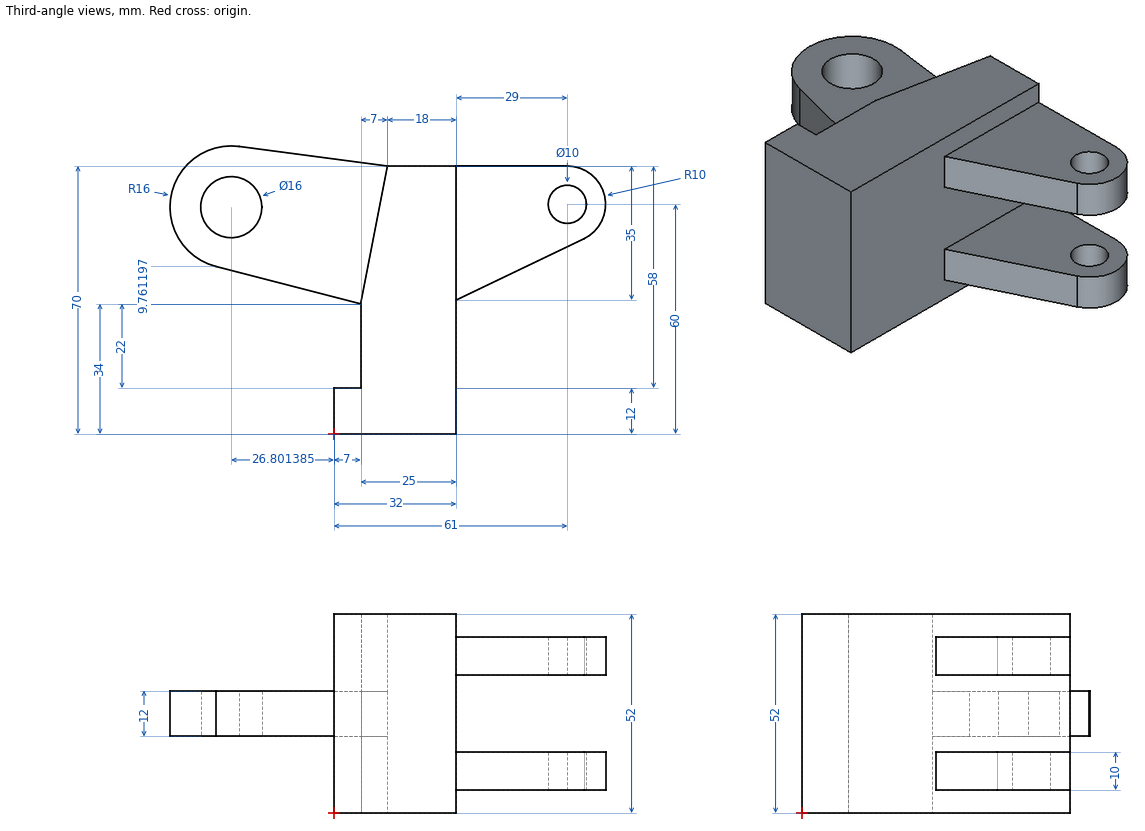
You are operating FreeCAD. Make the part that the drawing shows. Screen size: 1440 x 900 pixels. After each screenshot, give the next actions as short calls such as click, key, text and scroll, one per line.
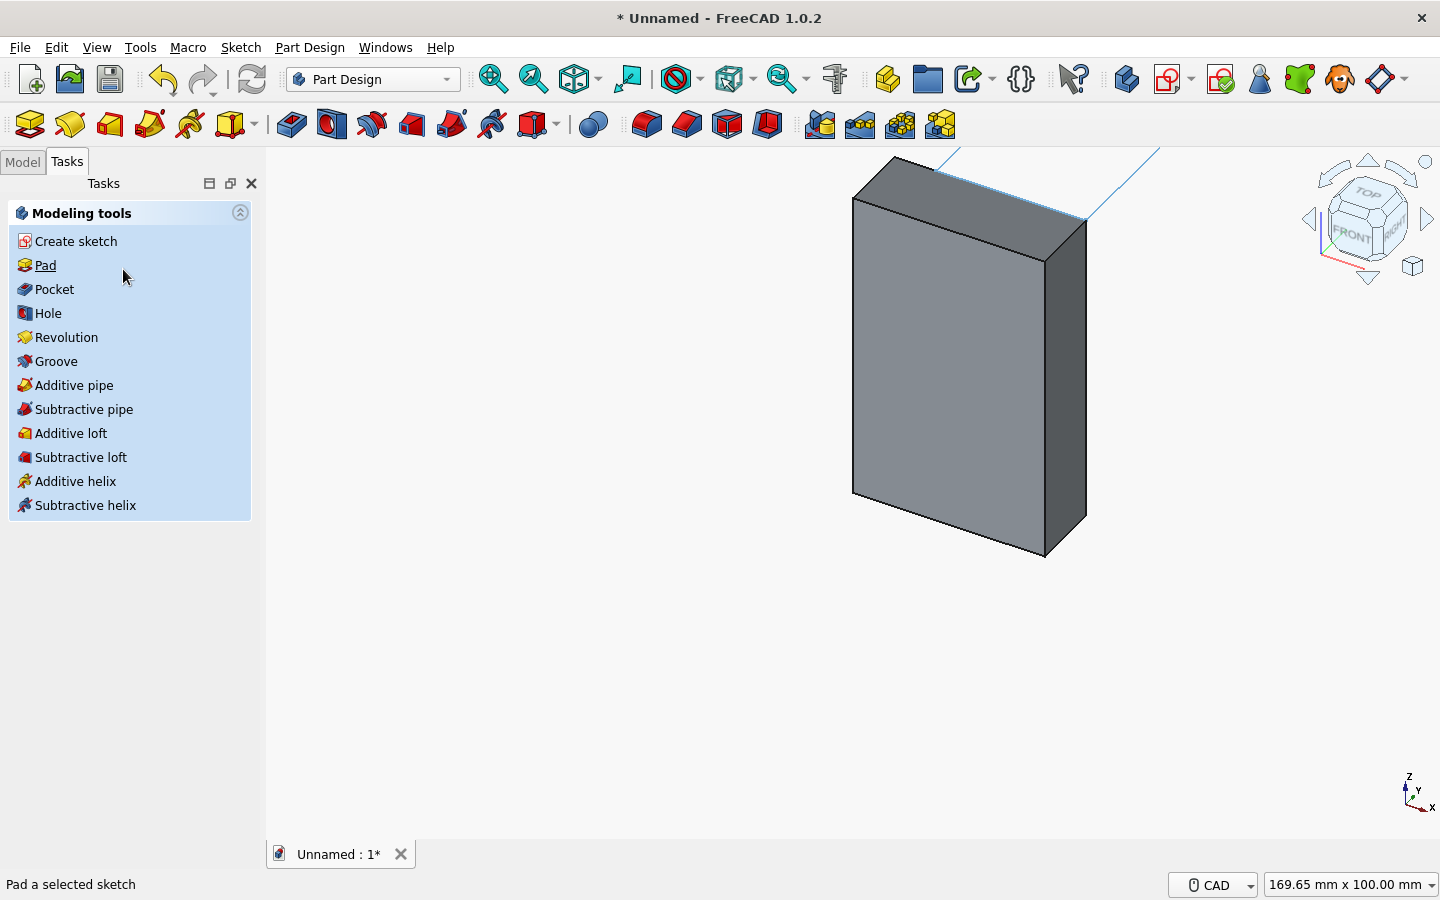
click(30, 124)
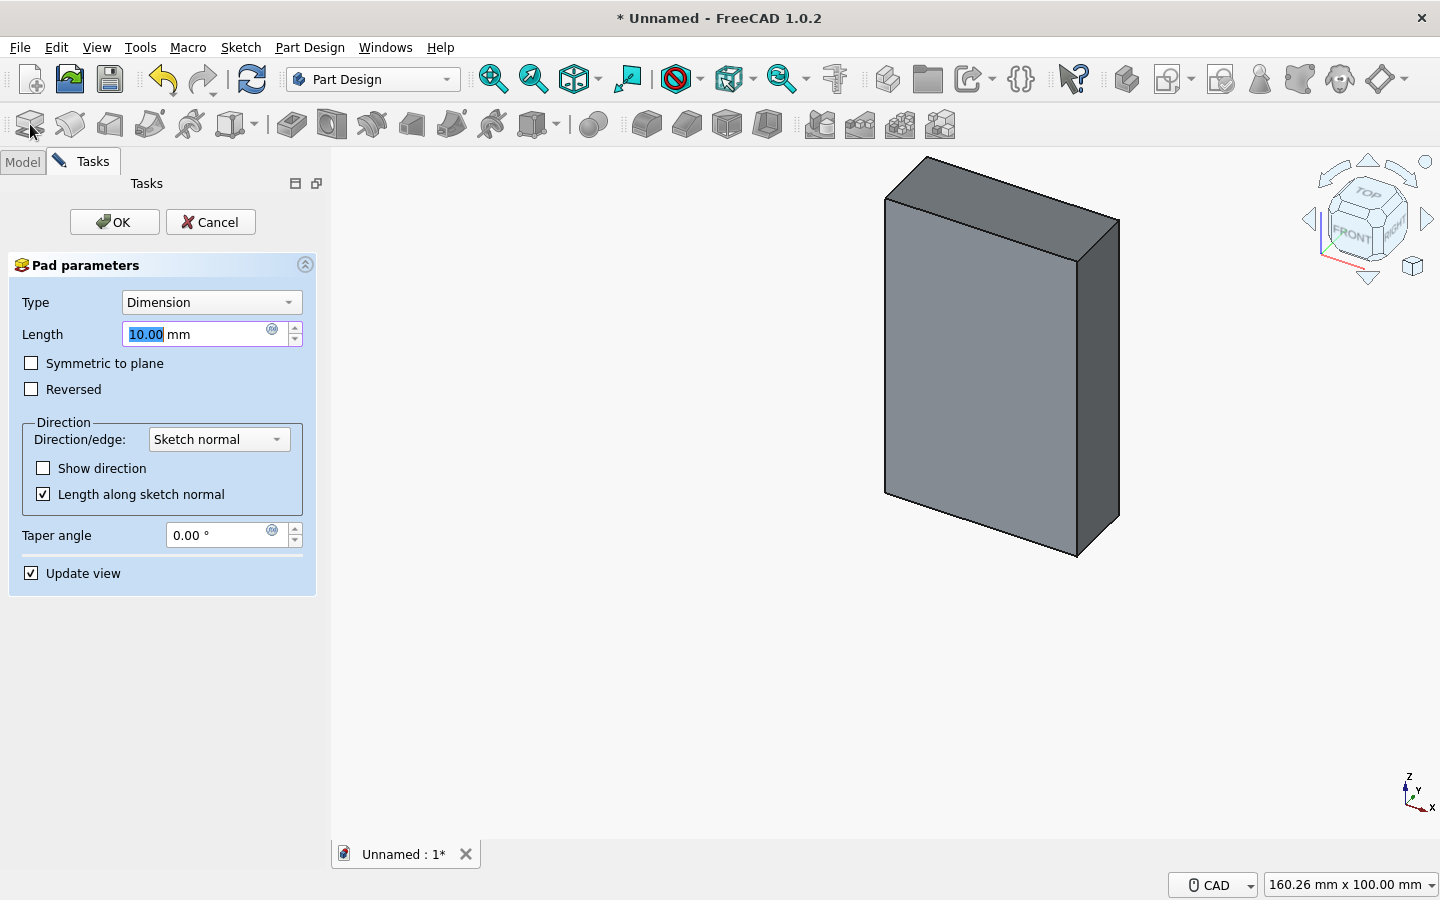
text(52)
key(Tab)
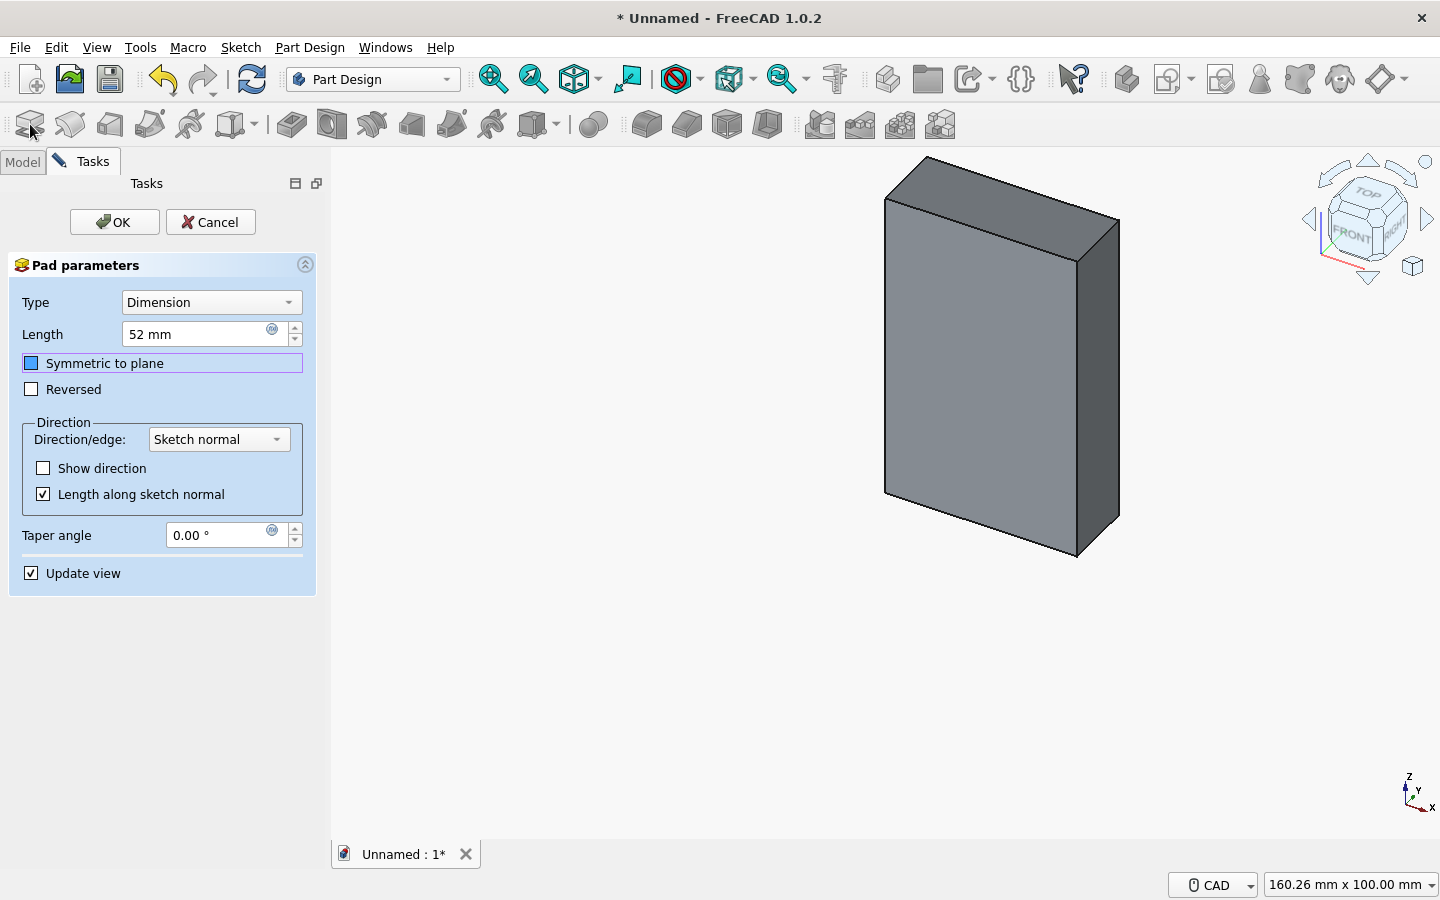
click(30, 389)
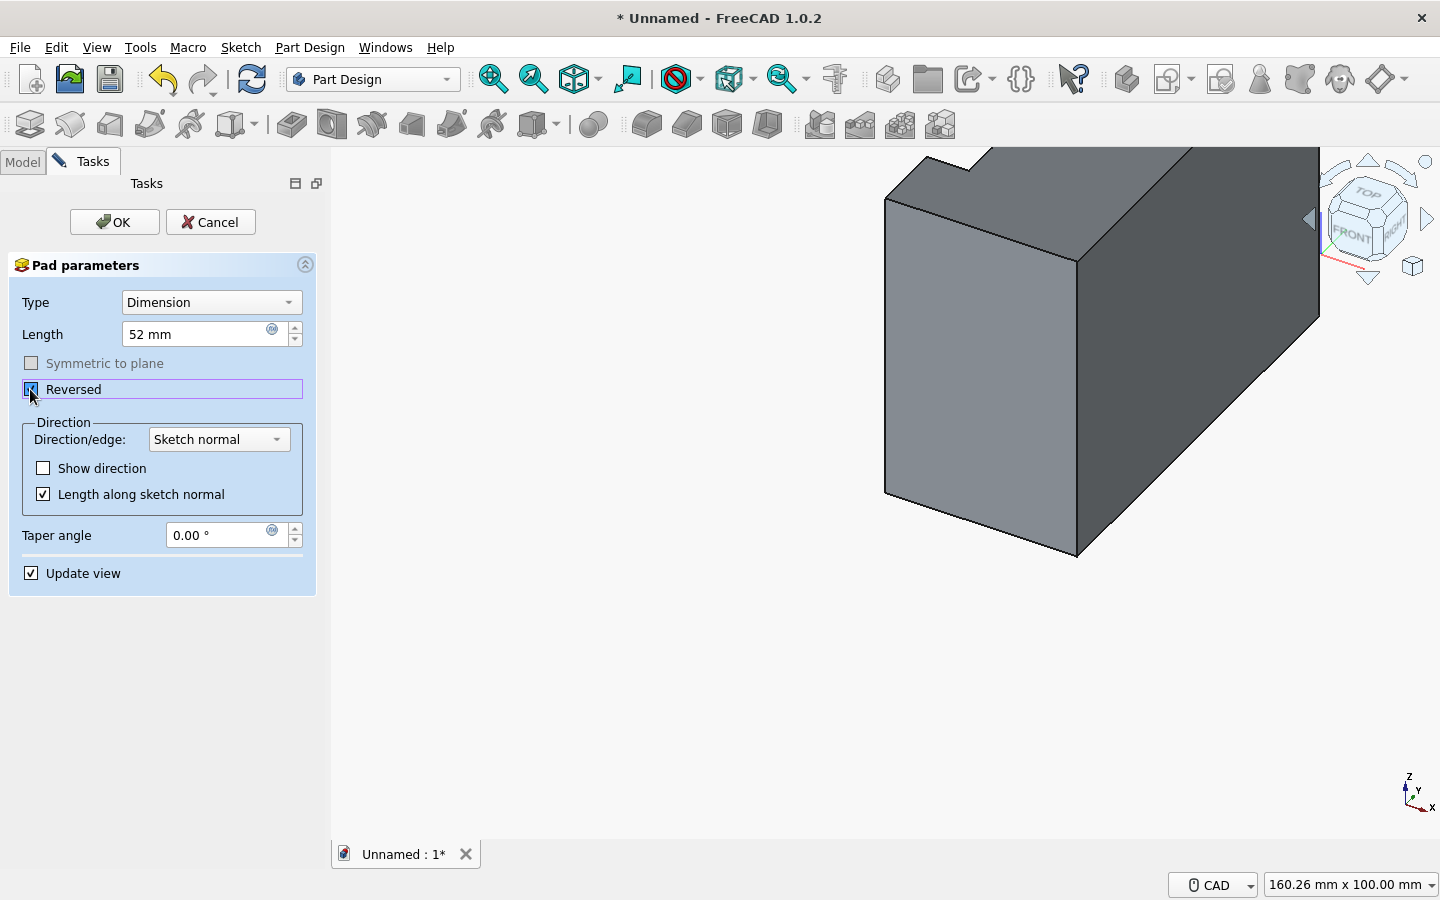
click(115, 222)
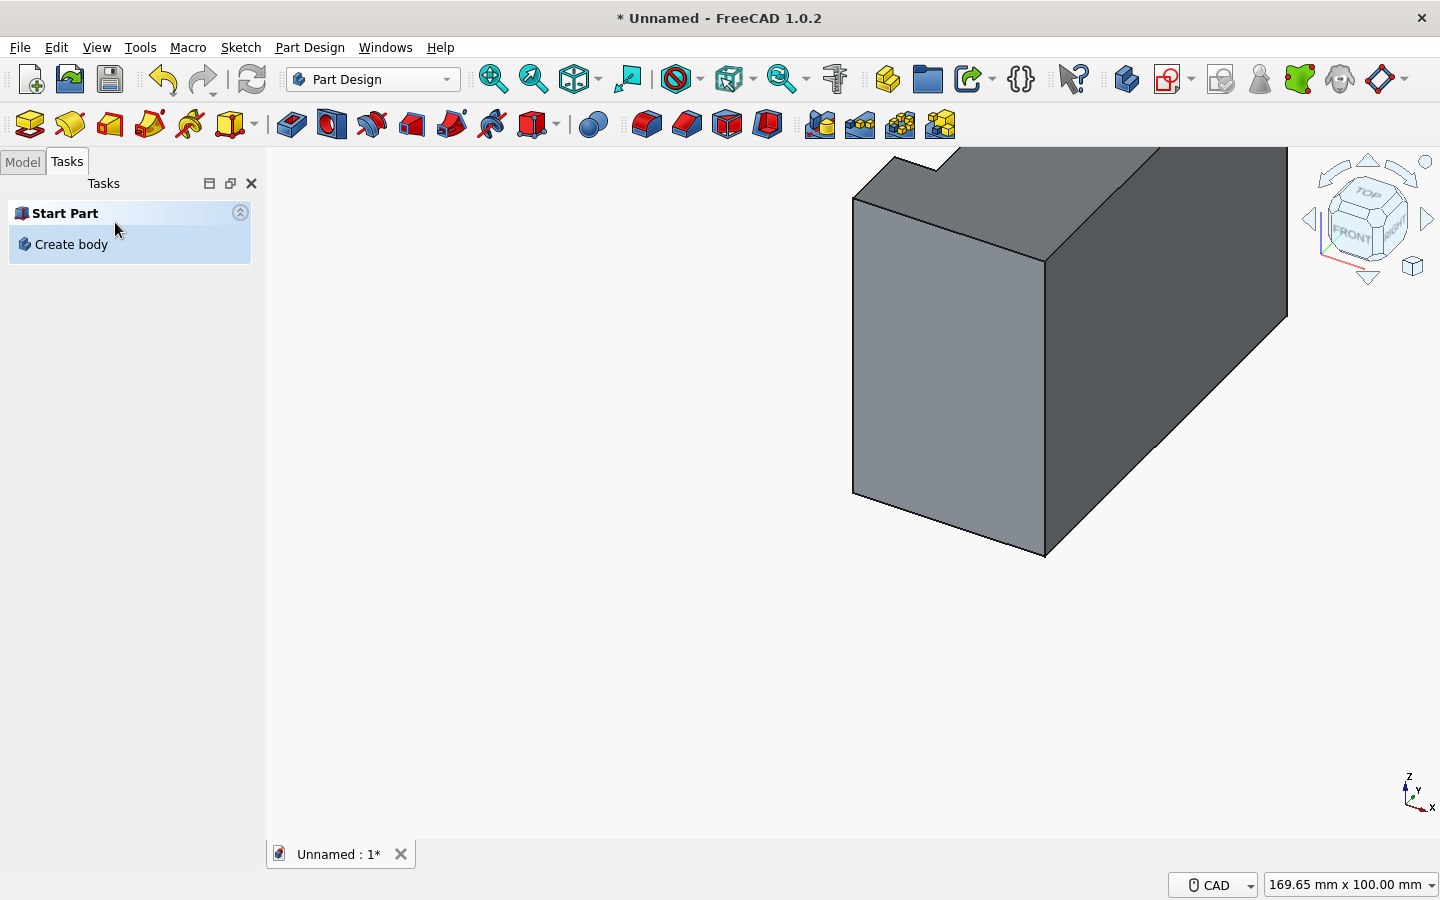
key(v)
key(f)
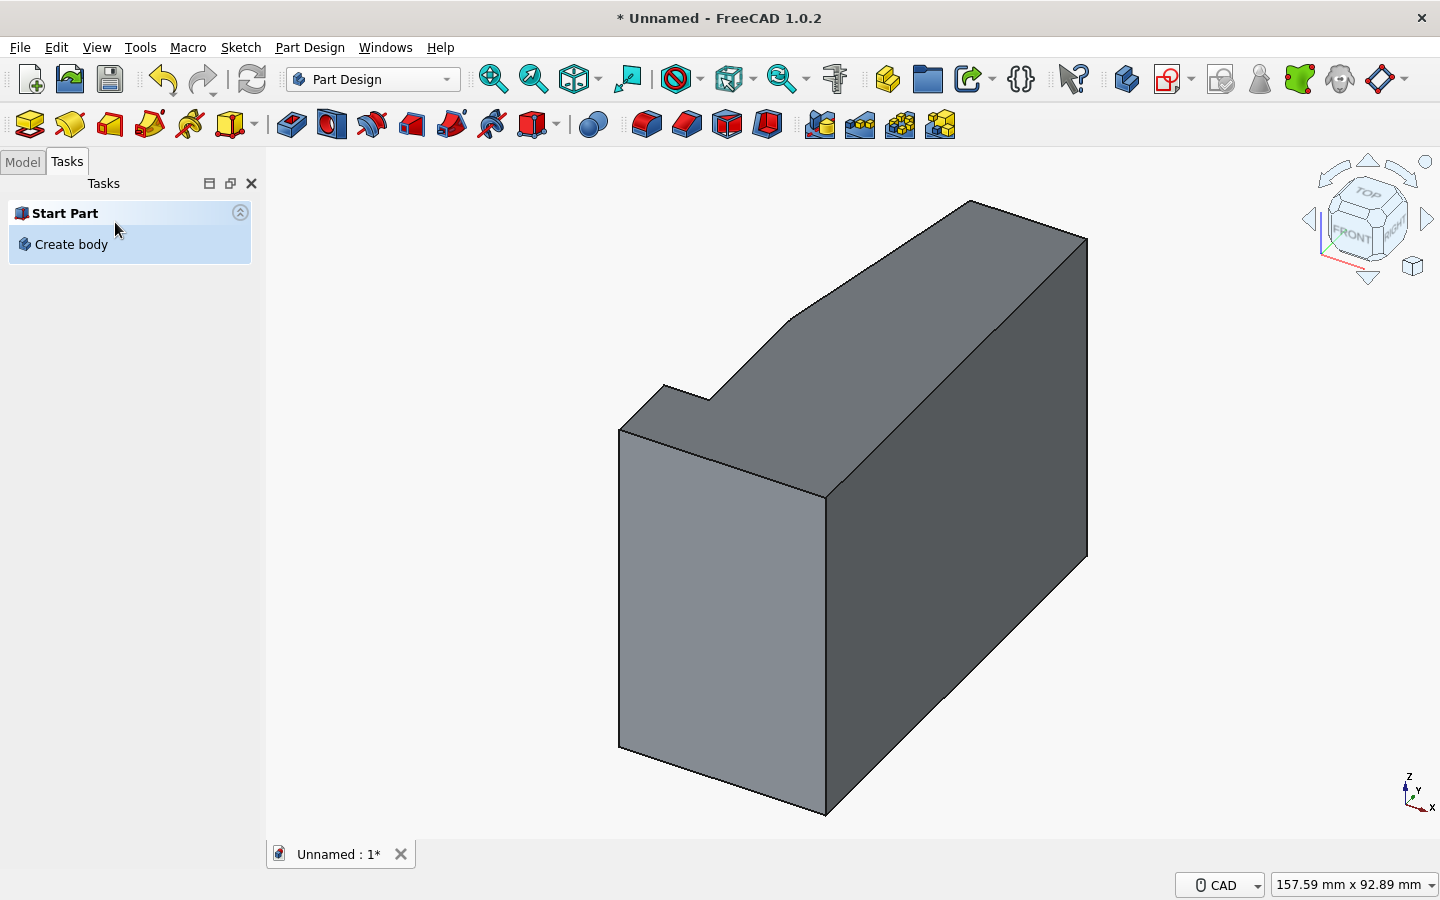
click(23, 161)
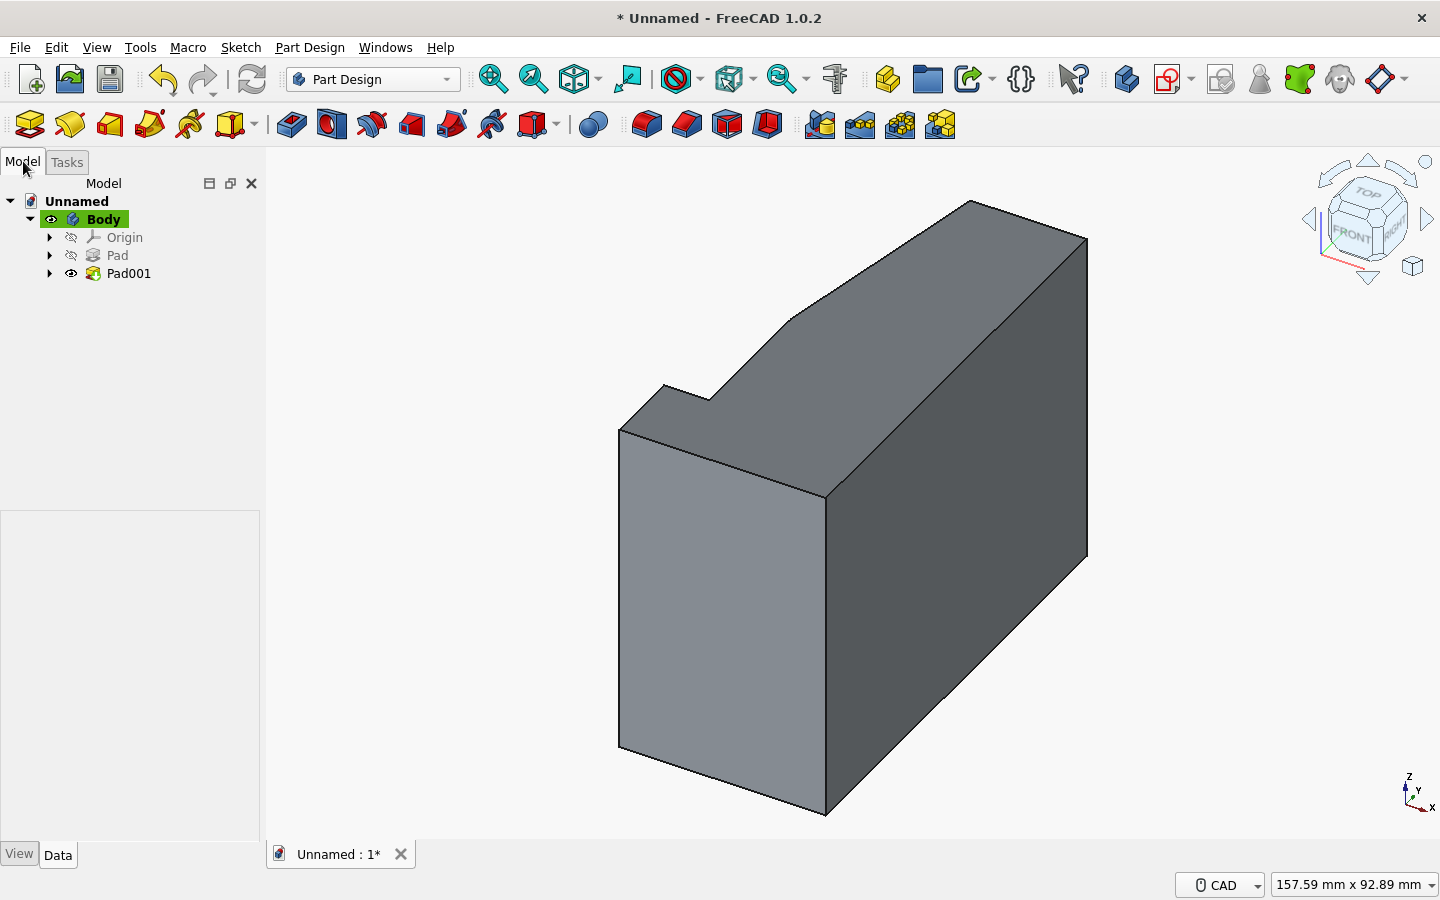
click(50, 237)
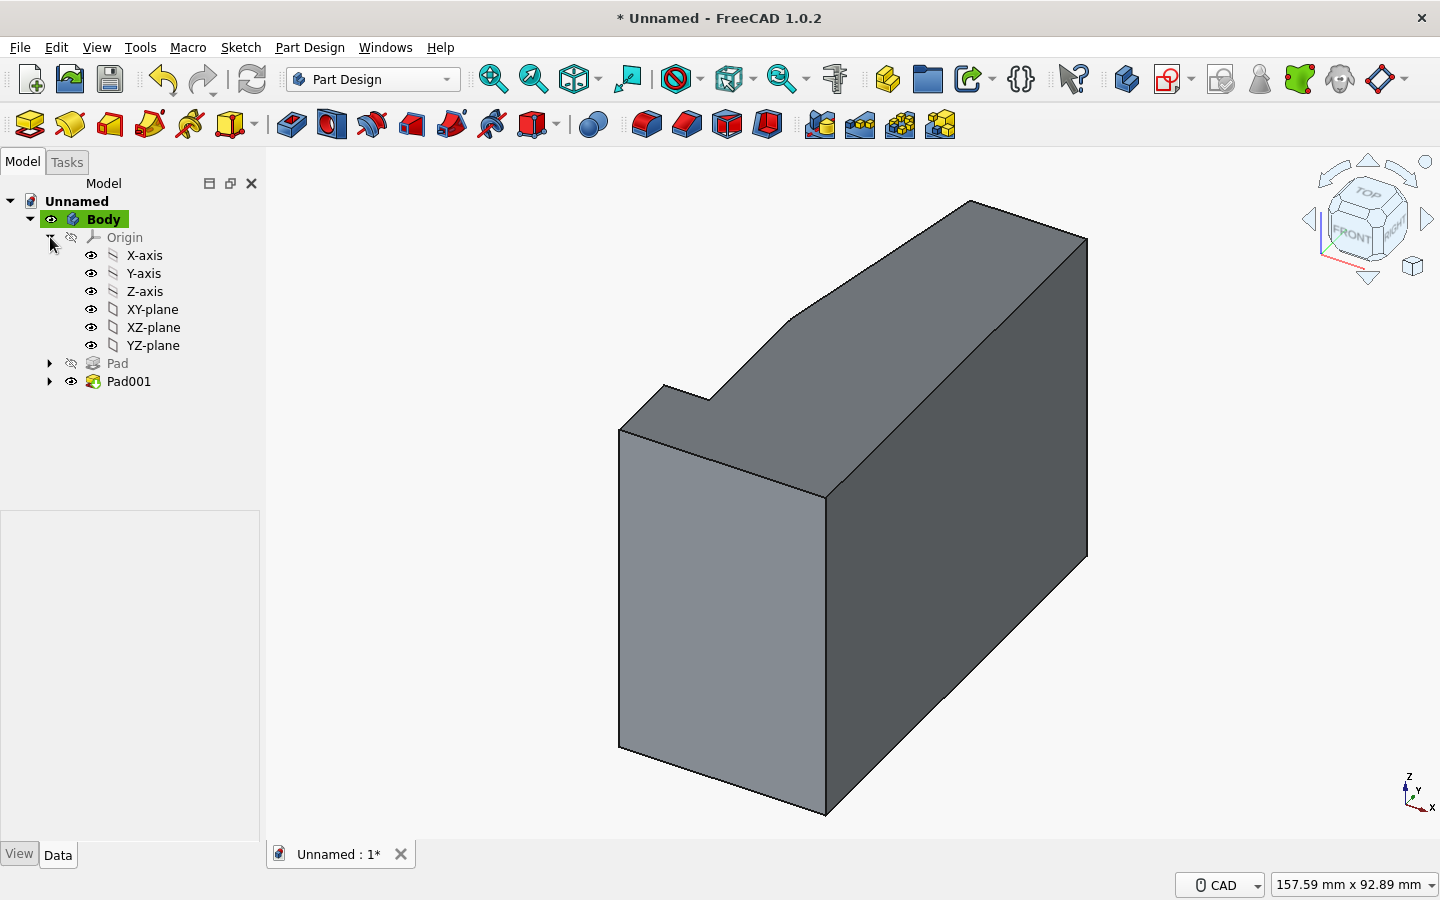
click(136, 309)